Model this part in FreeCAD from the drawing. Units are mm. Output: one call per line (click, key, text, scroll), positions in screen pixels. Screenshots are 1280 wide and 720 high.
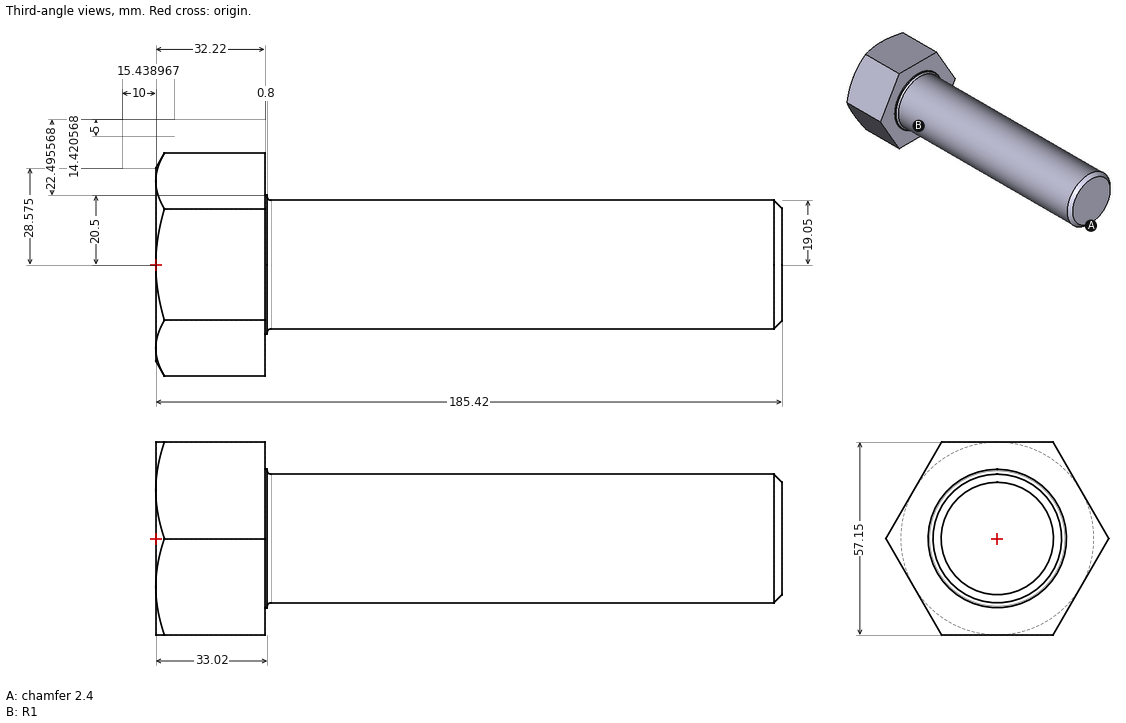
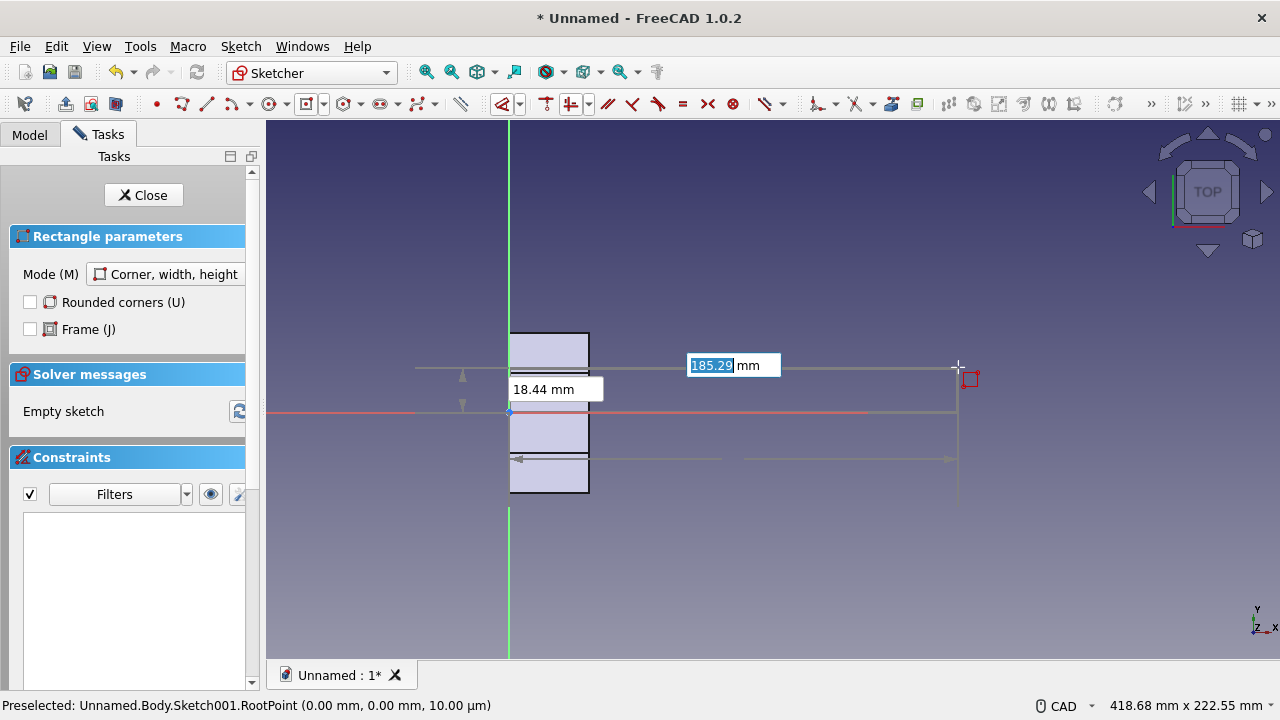
text(185.42)
key(Tab)
text(19.05)
key(Return)
key(Escape)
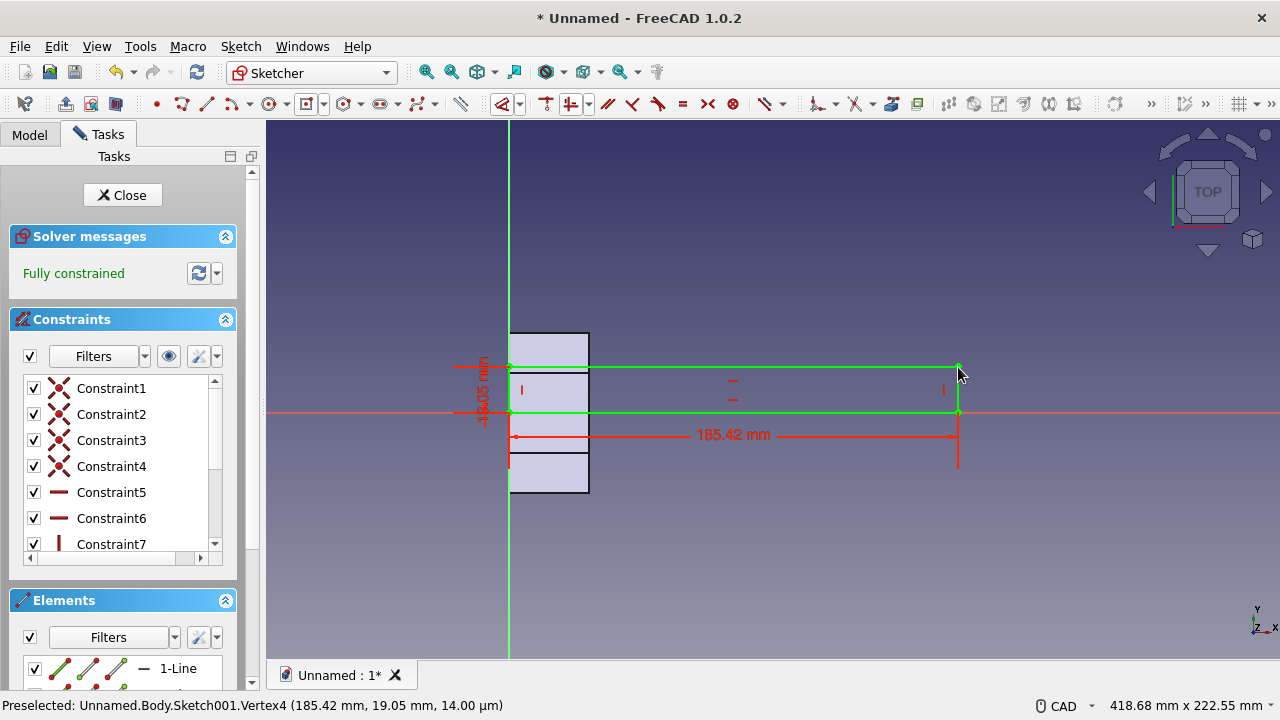
click(123, 195)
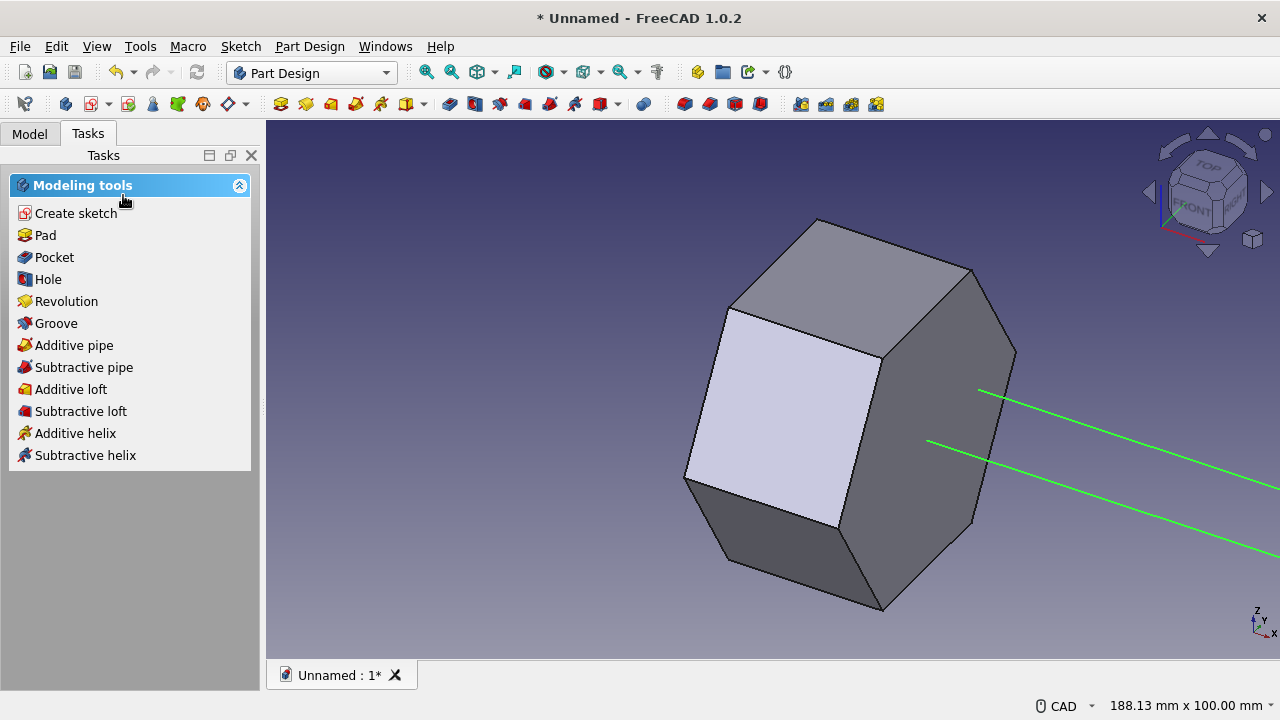
click(306, 104)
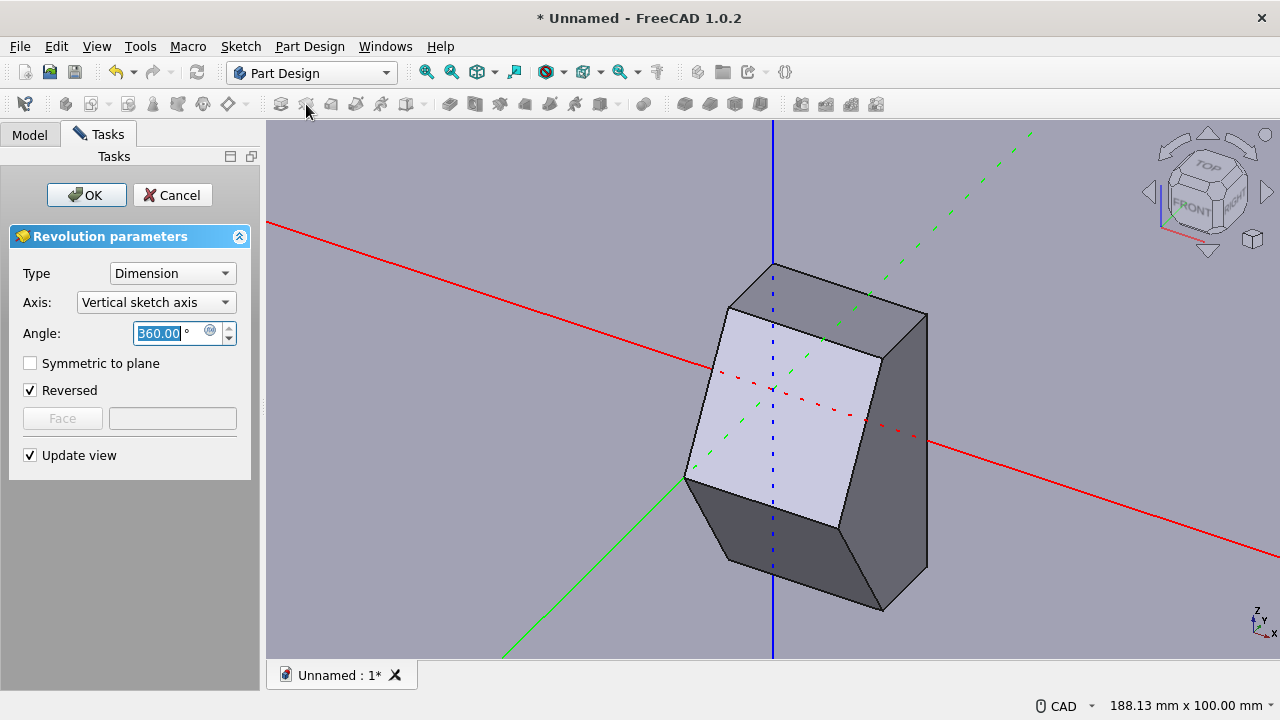
click(157, 302)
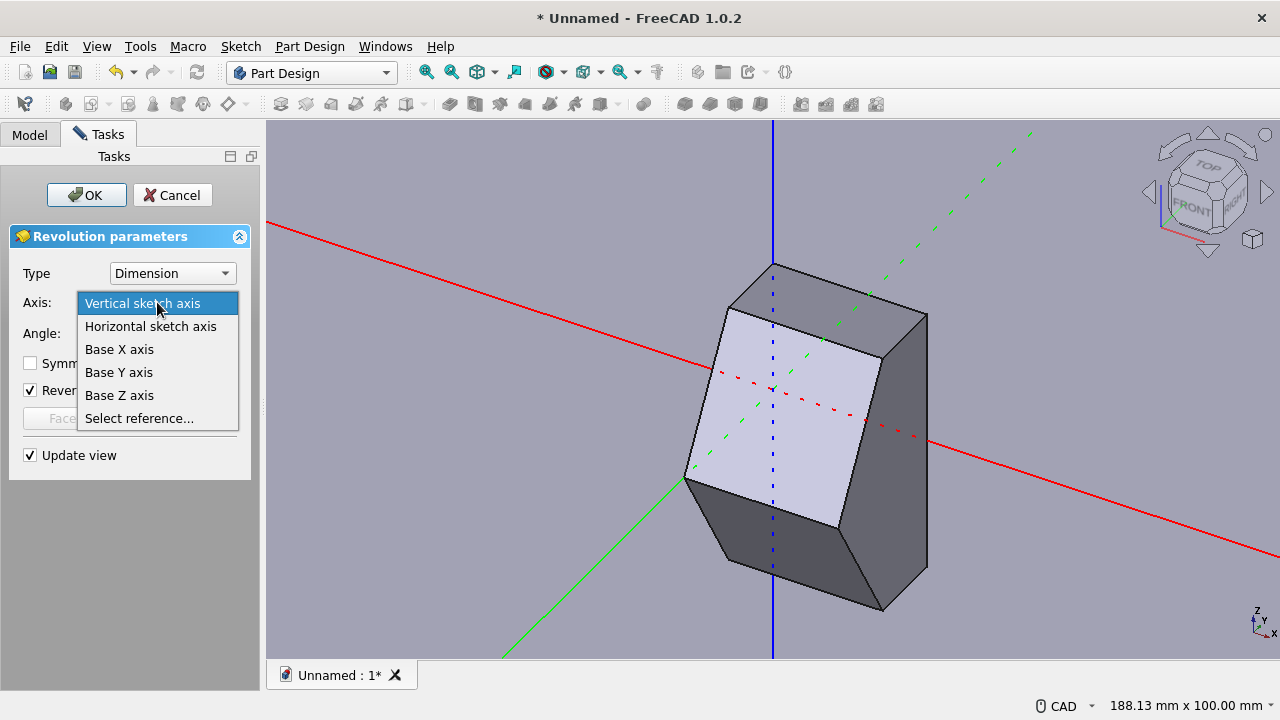
click(156, 326)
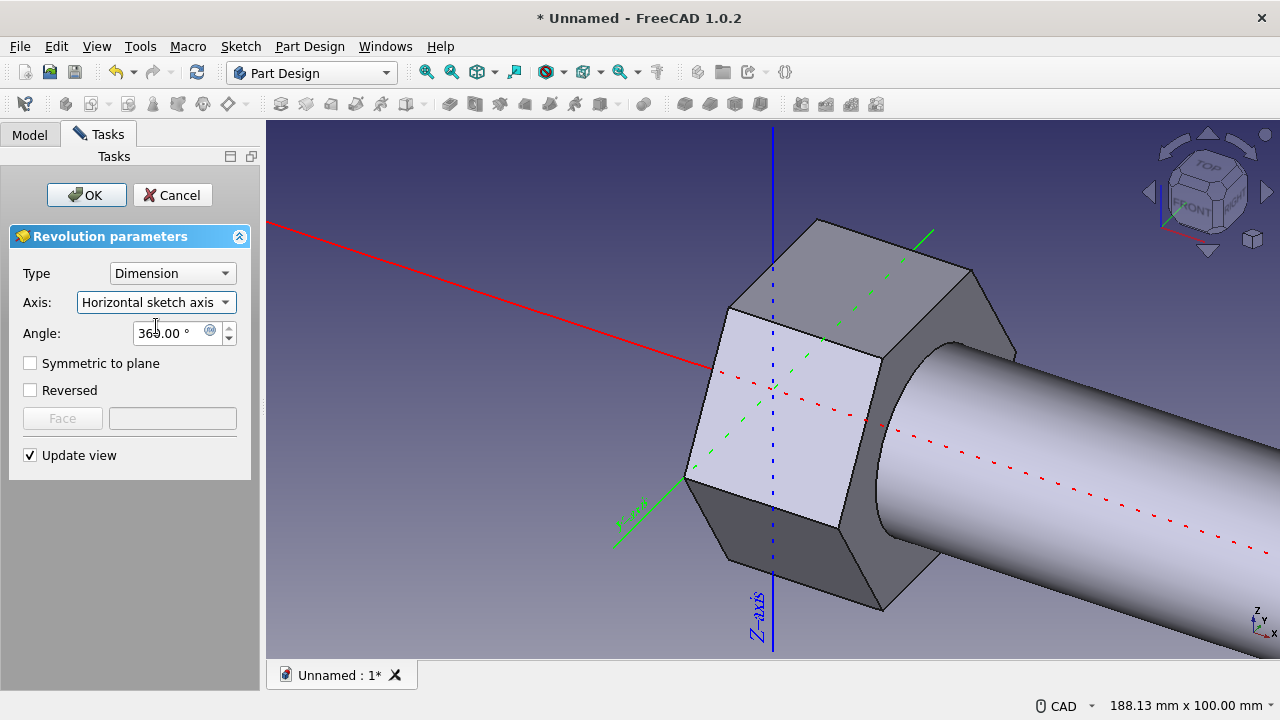
click(87, 195)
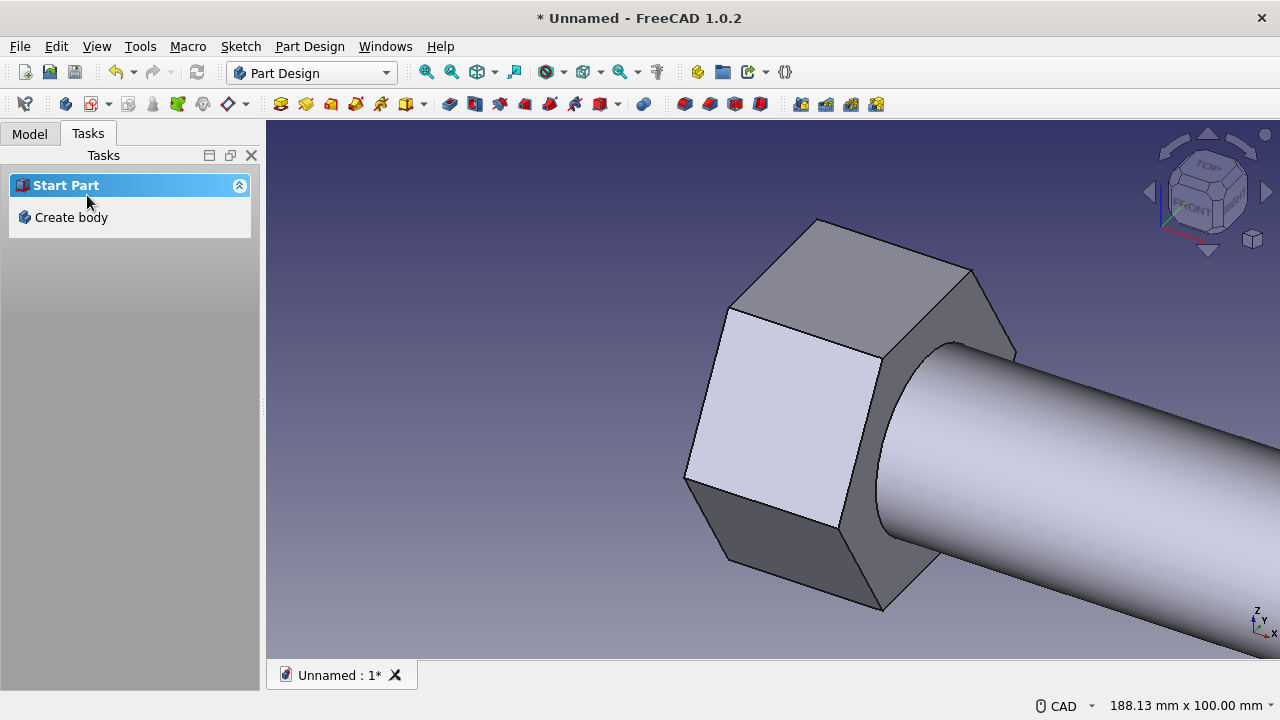
click(427, 72)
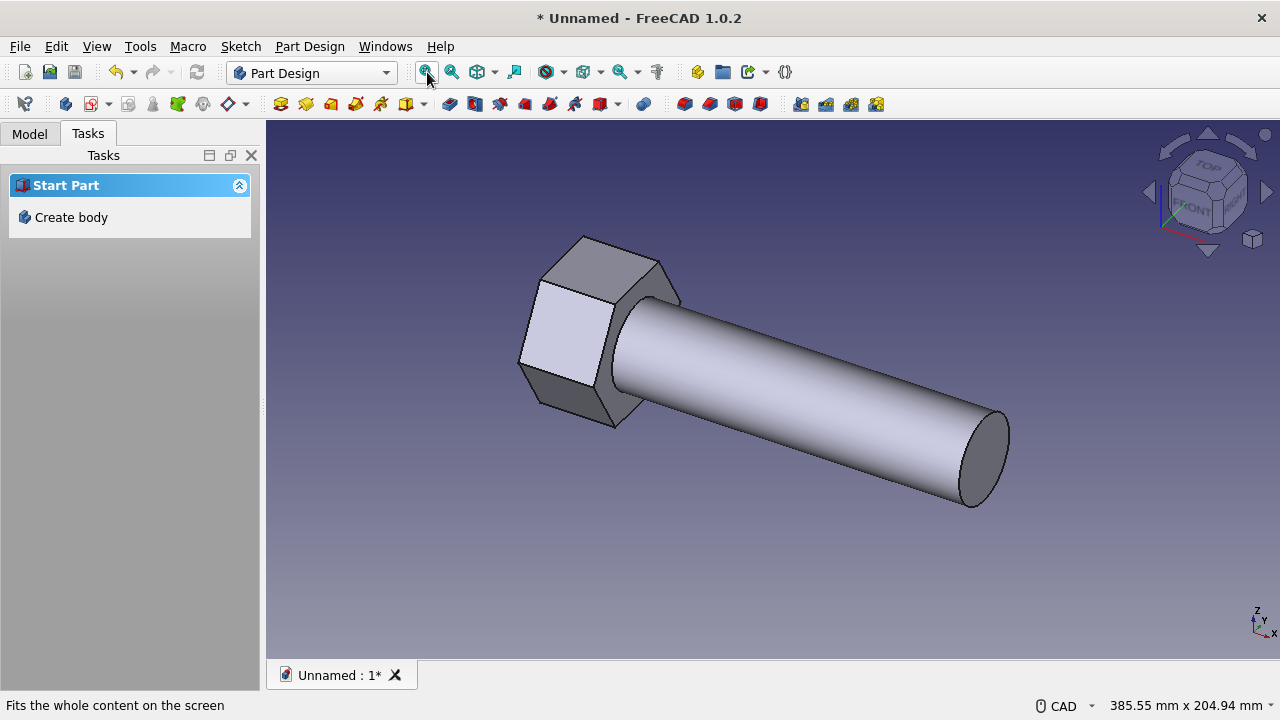
click(90, 104)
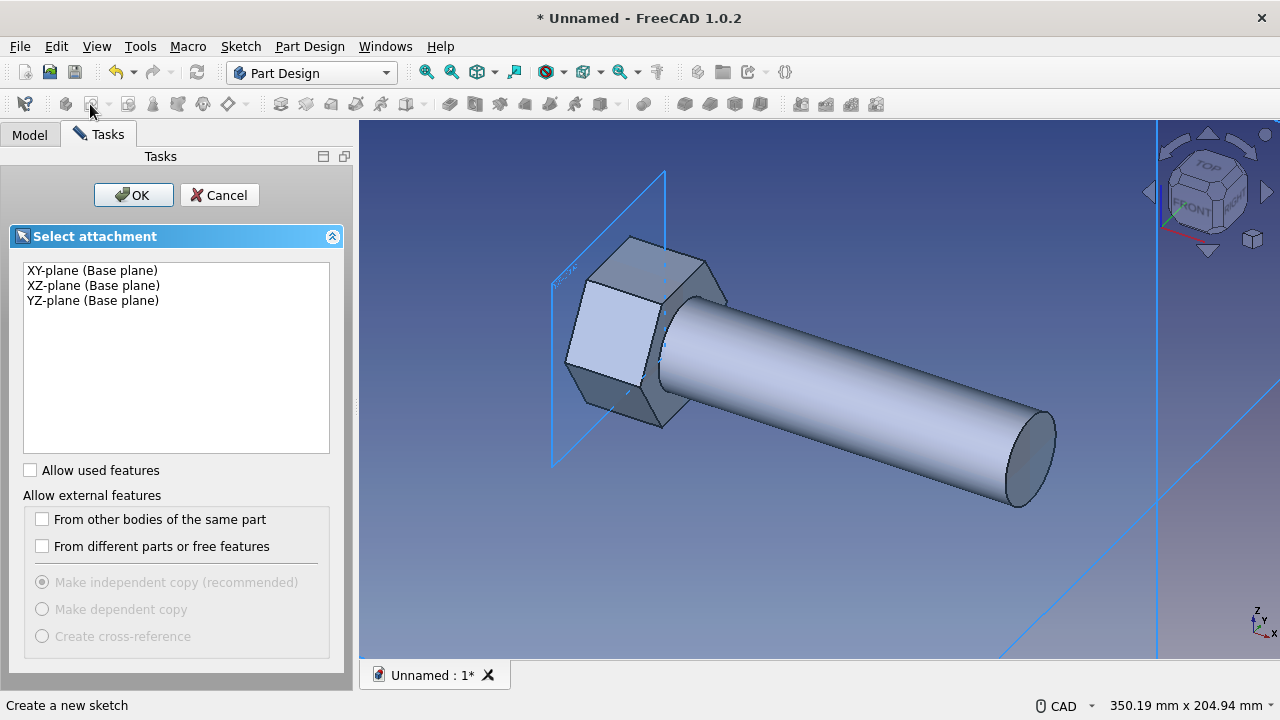
click(84, 270)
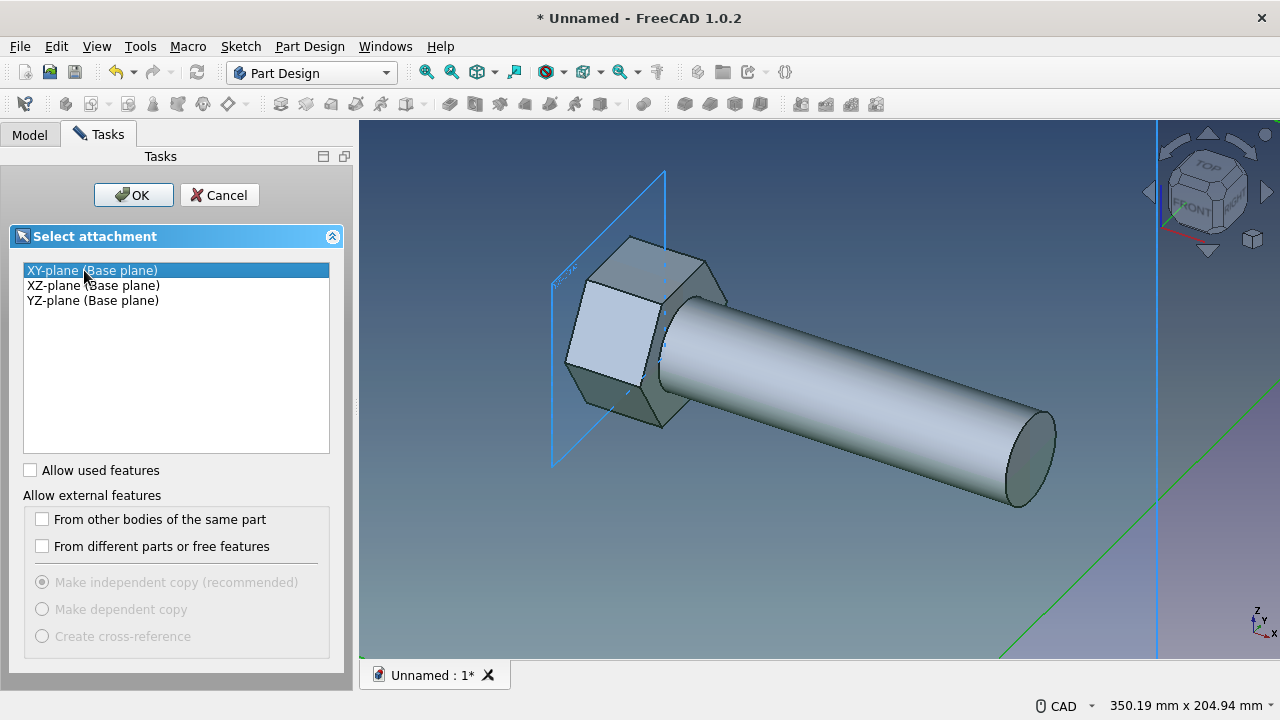
click(134, 195)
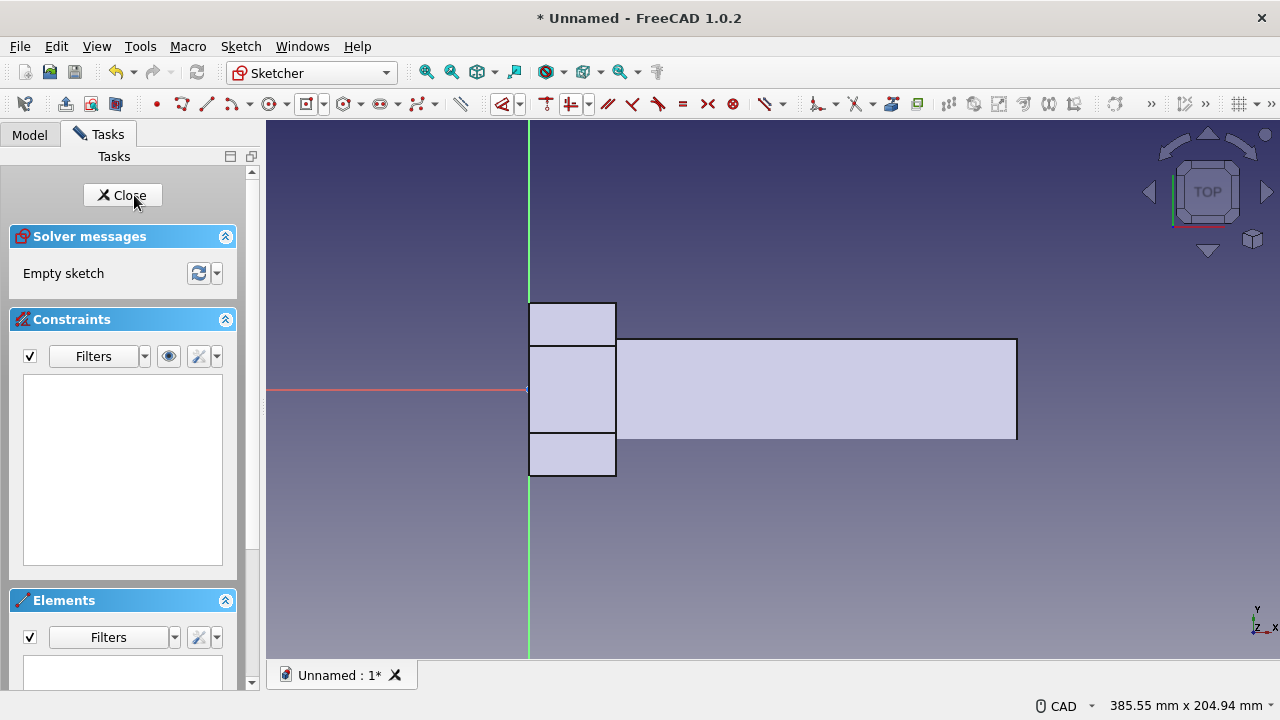
click(116, 104)